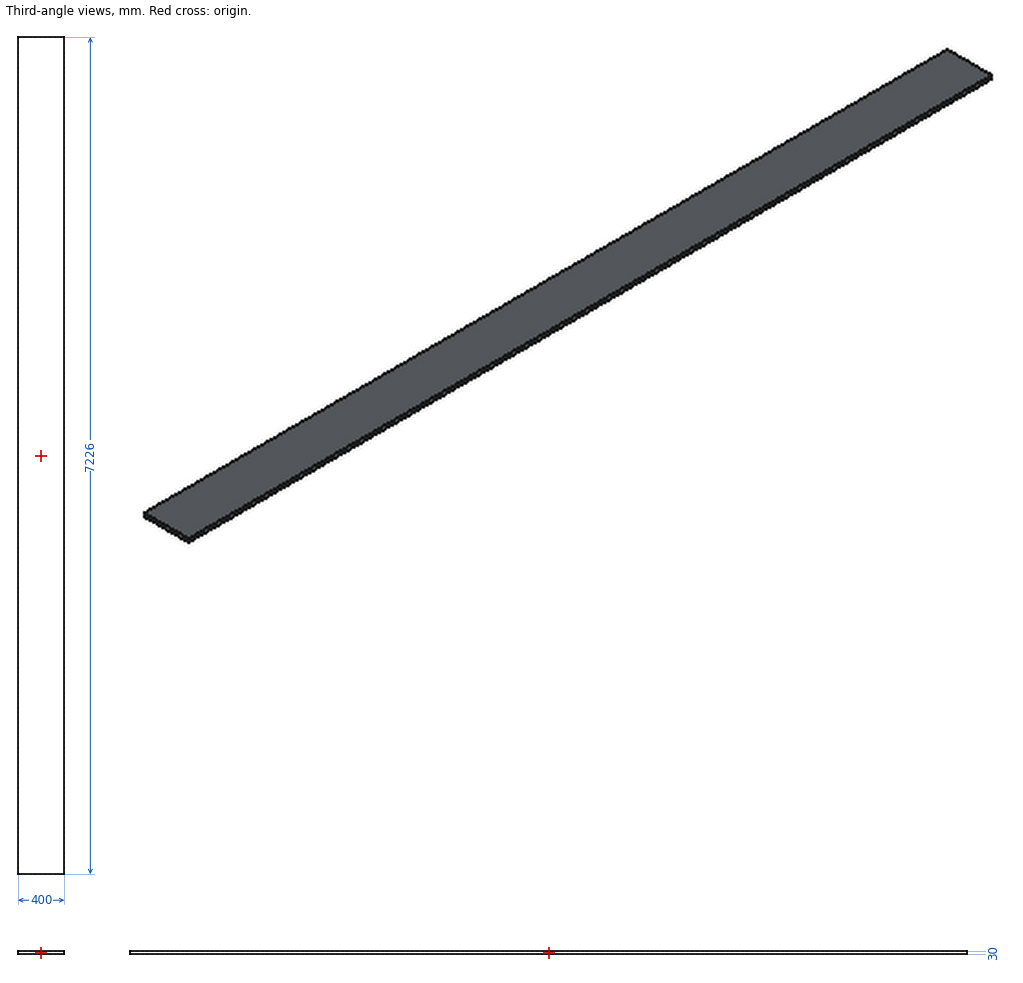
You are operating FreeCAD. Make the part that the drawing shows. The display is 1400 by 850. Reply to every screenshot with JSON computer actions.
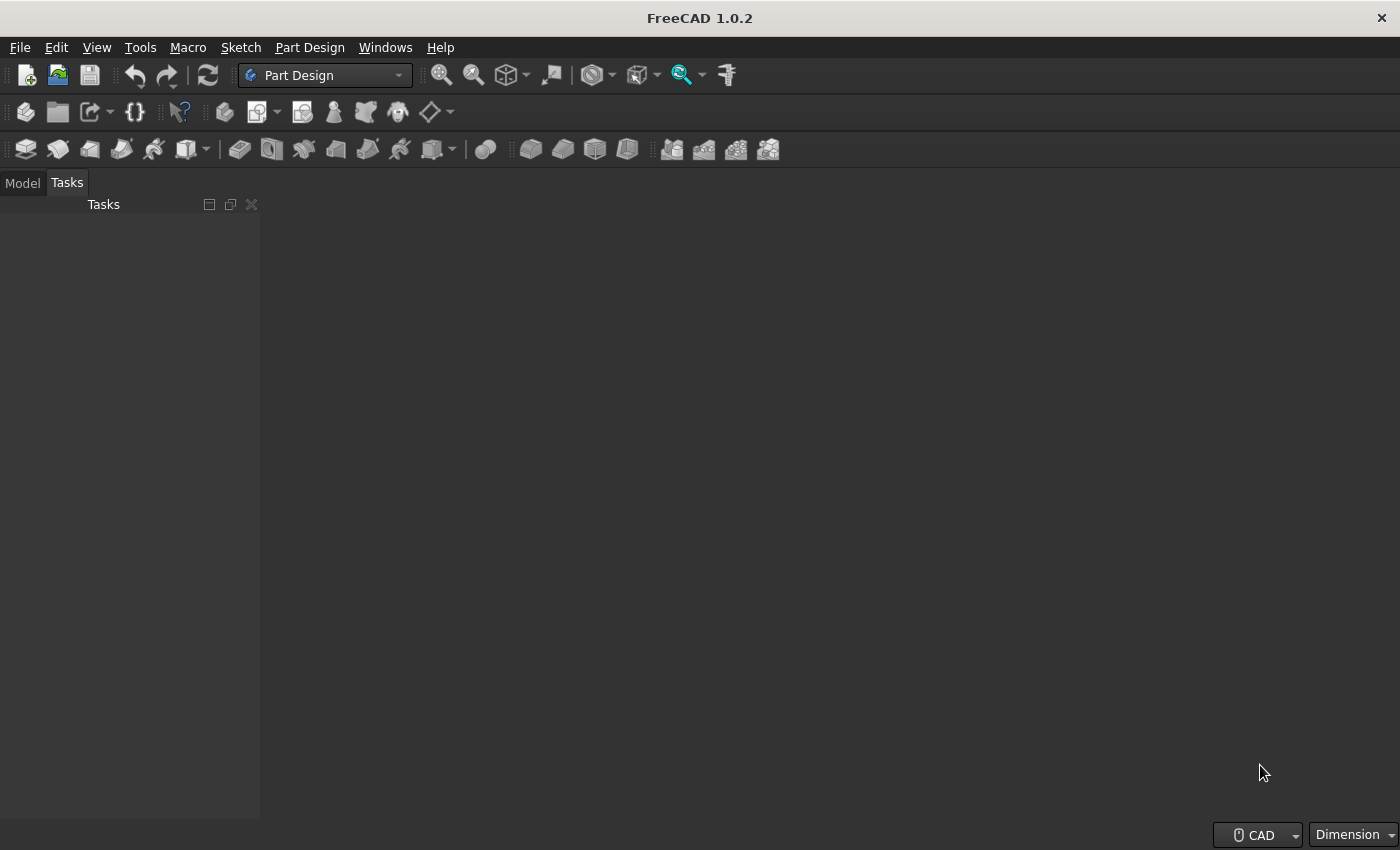
{"action": "left_click", "coordinate": [26, 76]}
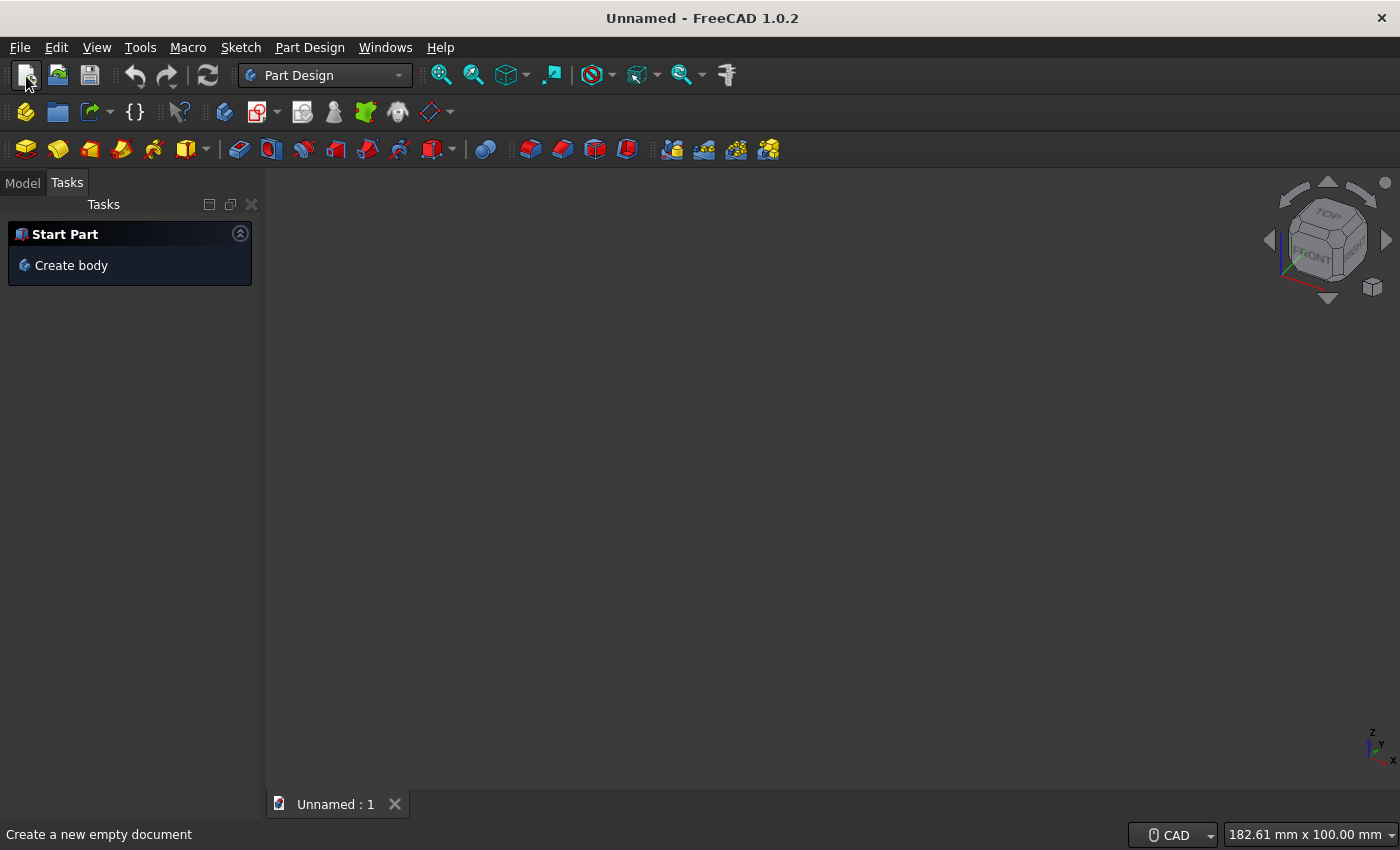
{"action": "left_click", "coordinate": [258, 112]}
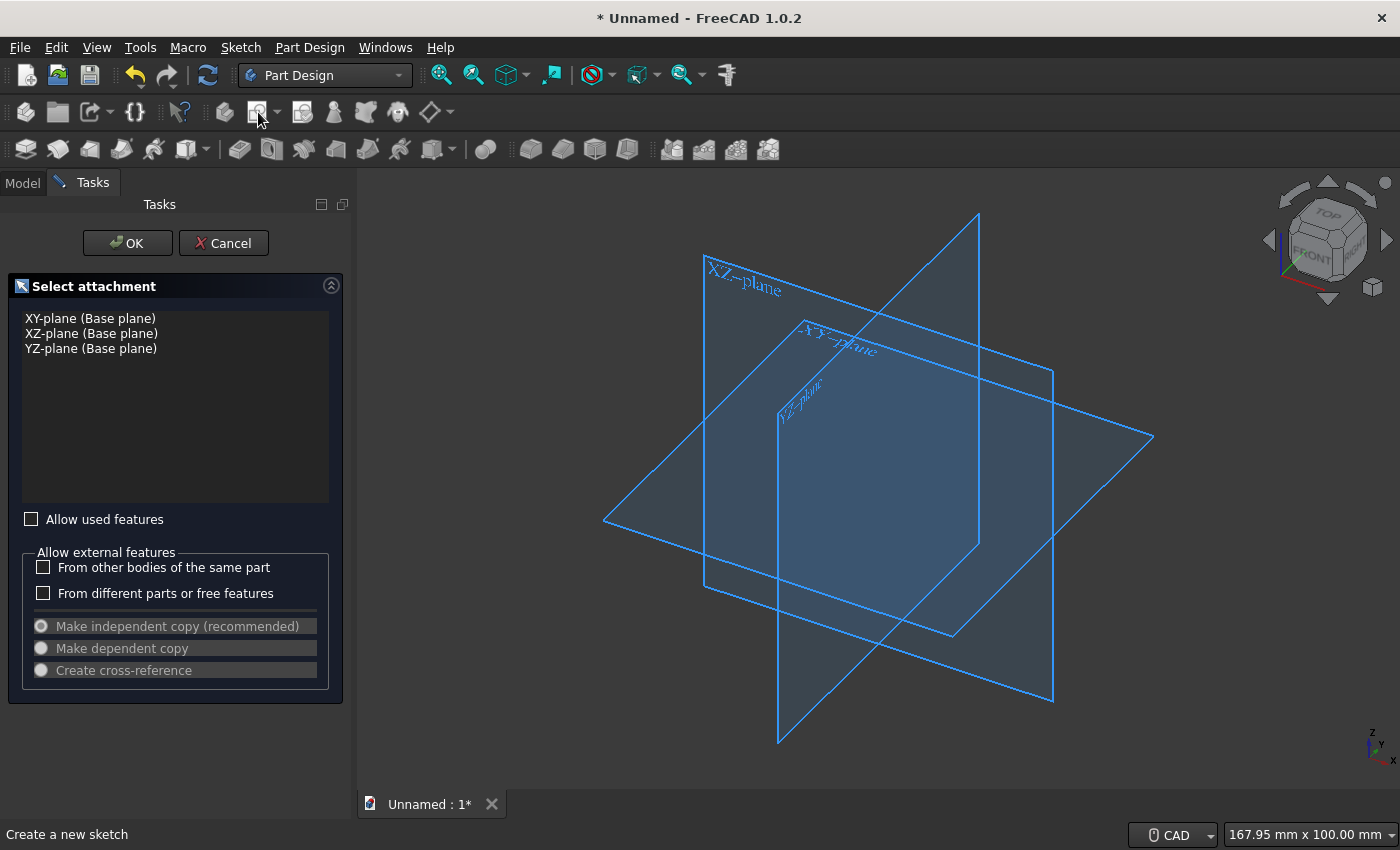
{"action": "left_click", "coordinate": [82, 318]}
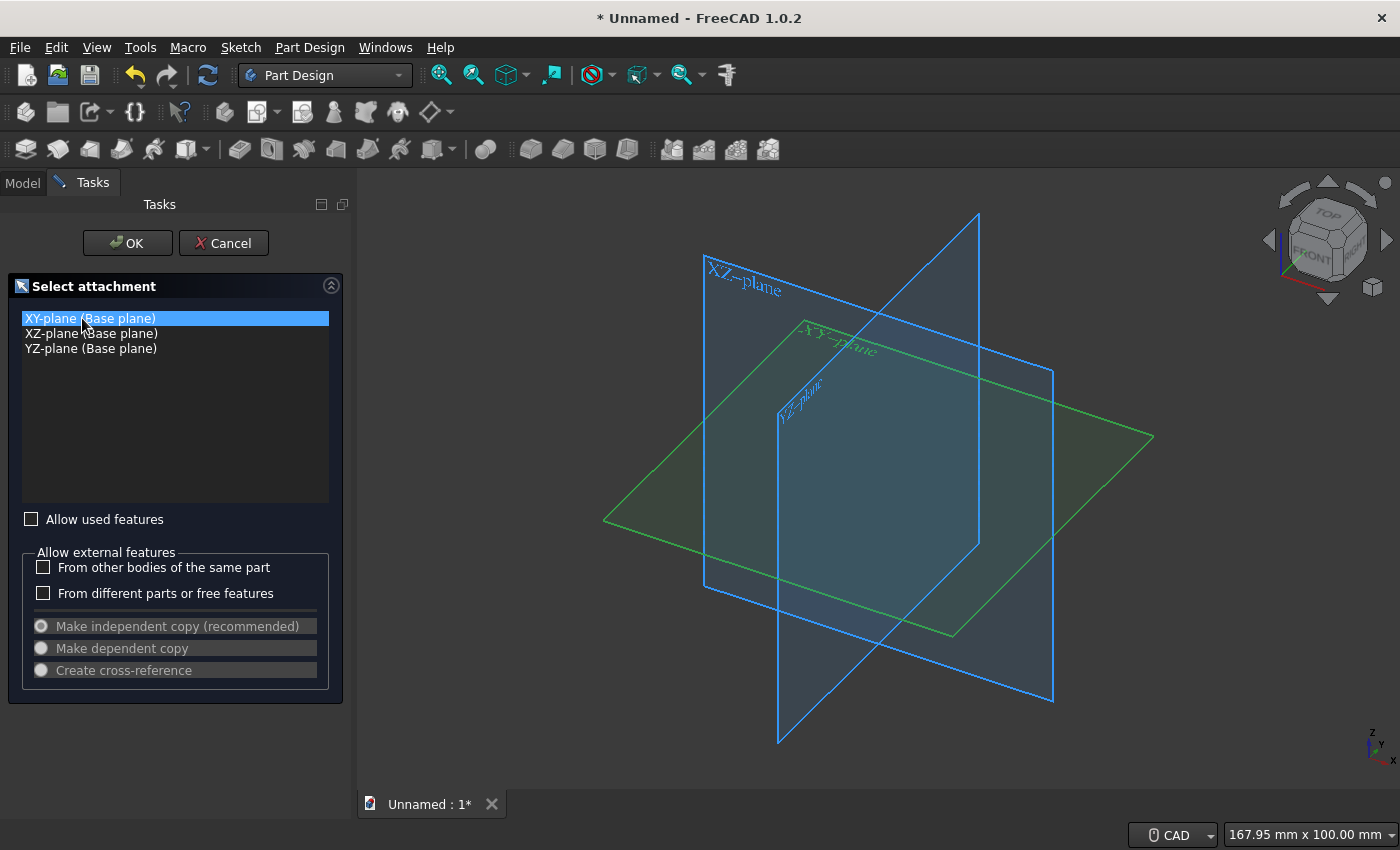
{"action": "left_click", "coordinate": [128, 243]}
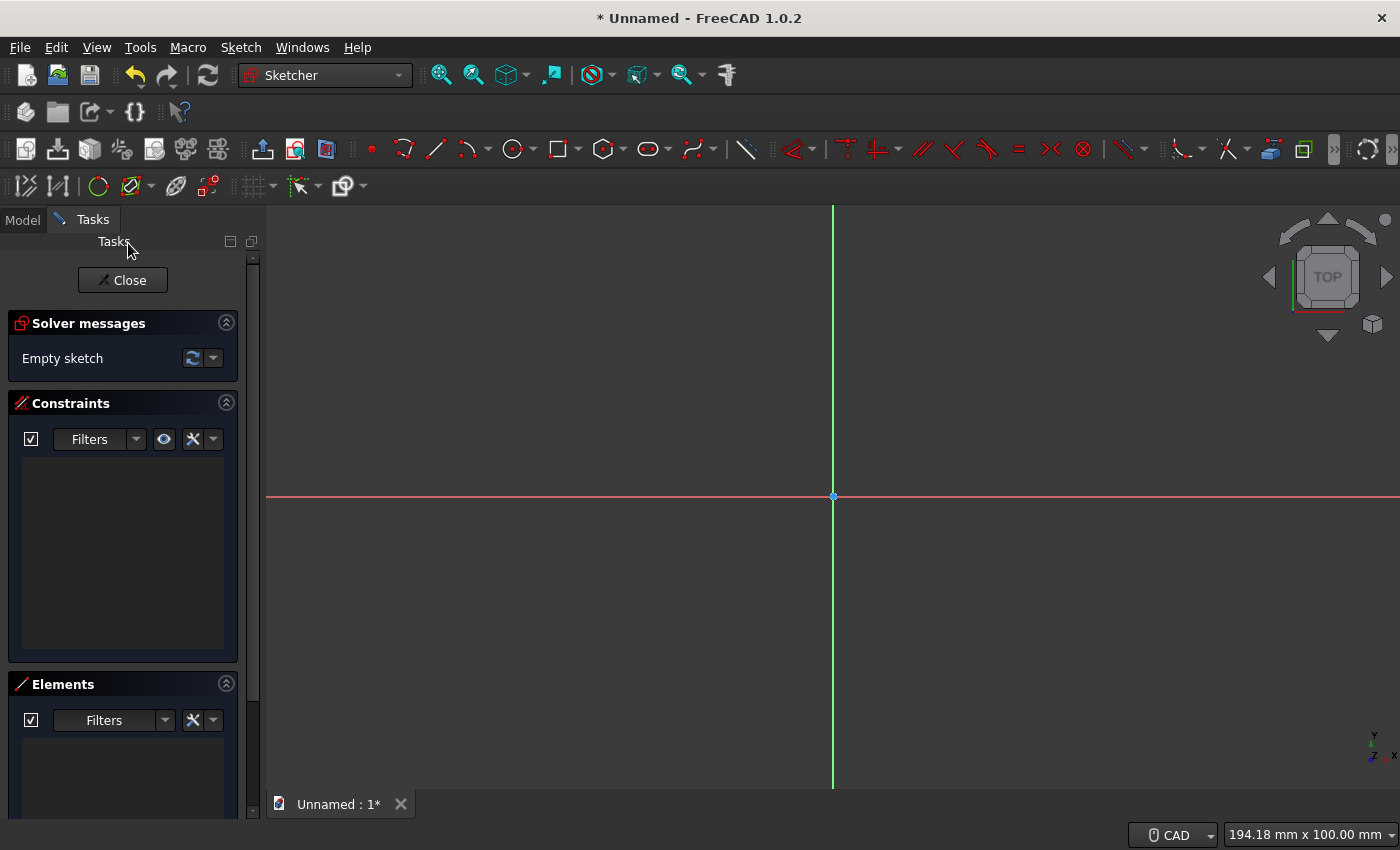
{"action": "scroll", "coordinate": [764, 497], "scroll_direction": "down", "scroll_amount": 15}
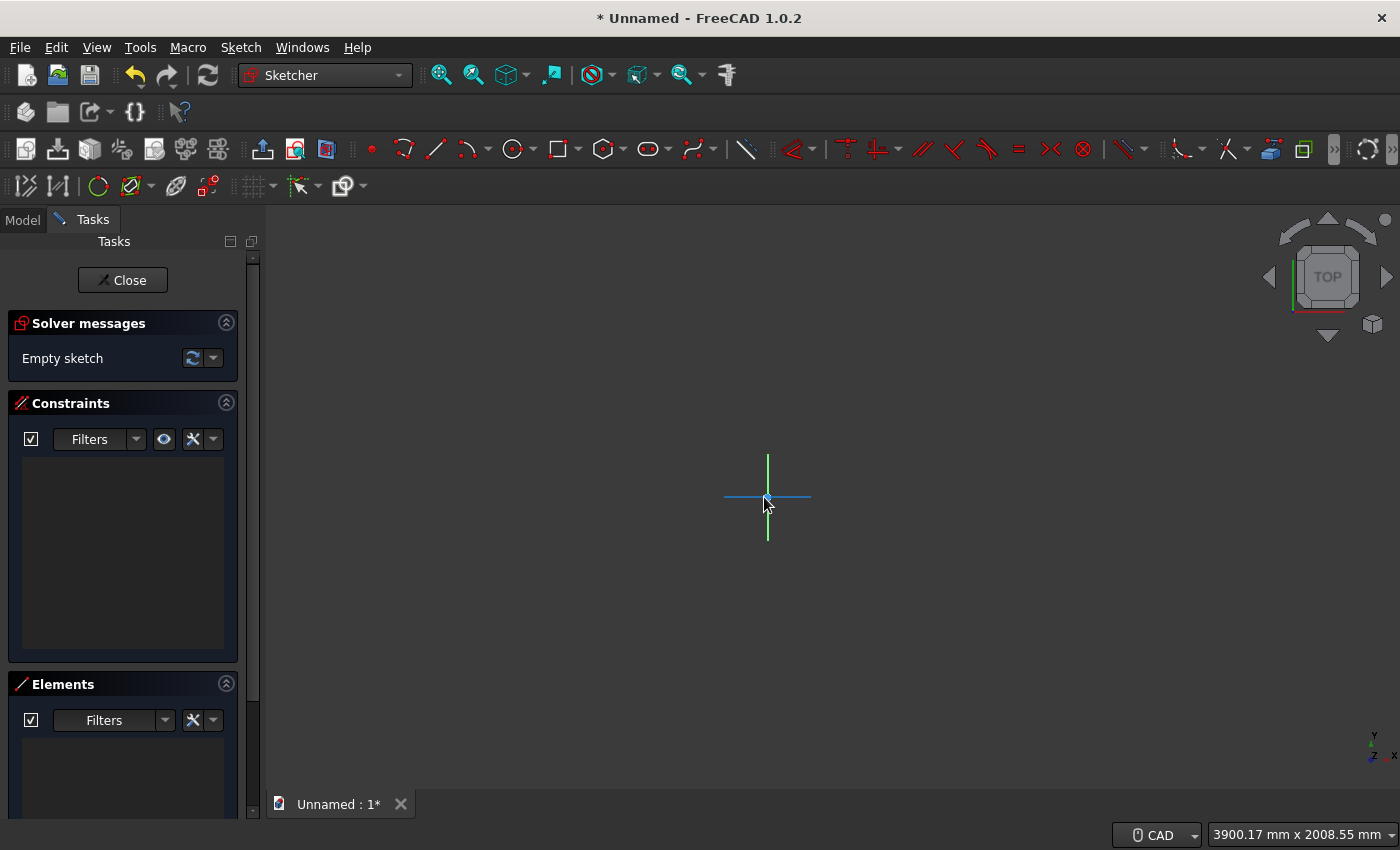
{"action": "scroll", "coordinate": [764, 497], "scroll_direction": "down", "scroll_amount": 9}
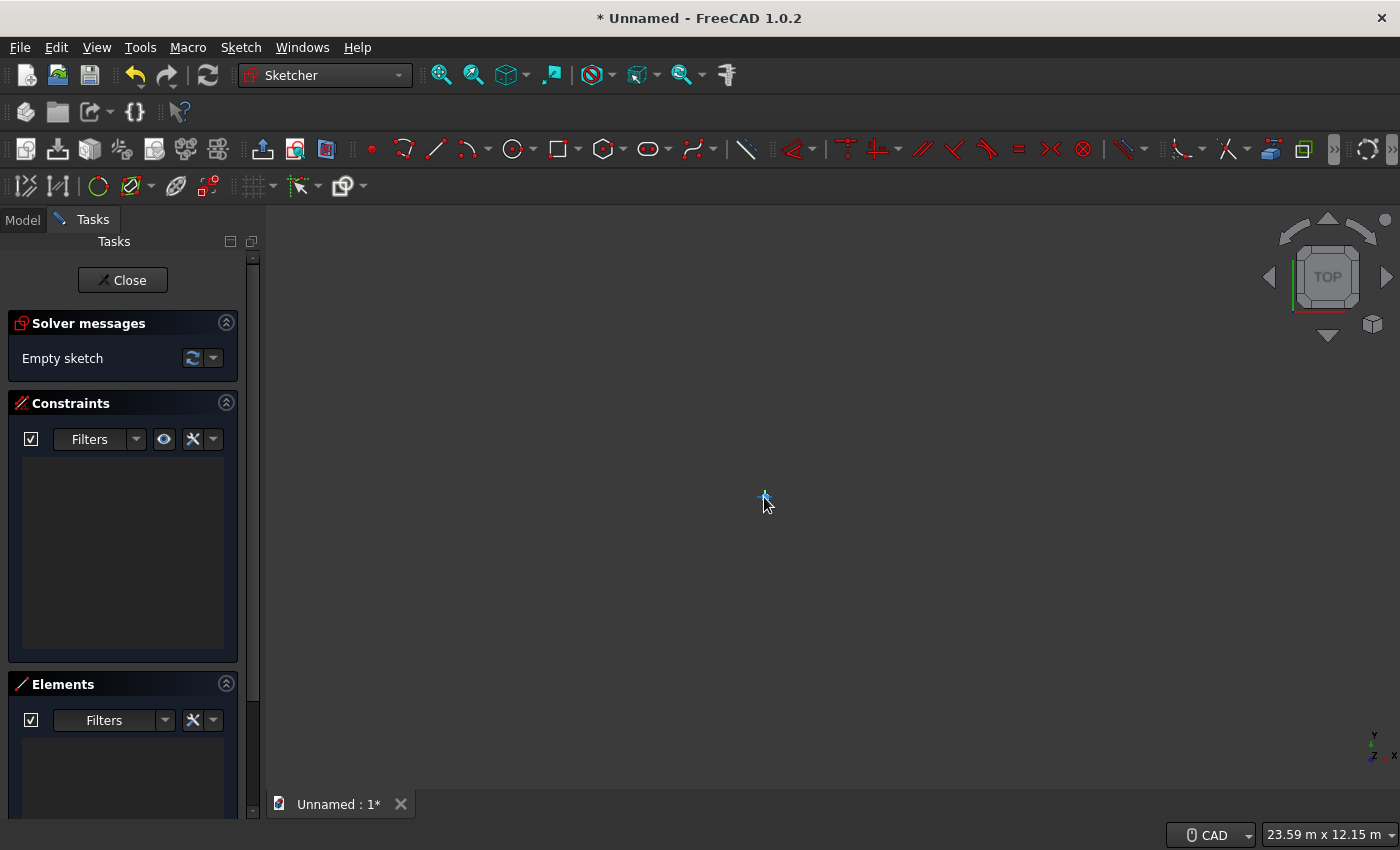
{"action": "left_click", "coordinate": [580, 150]}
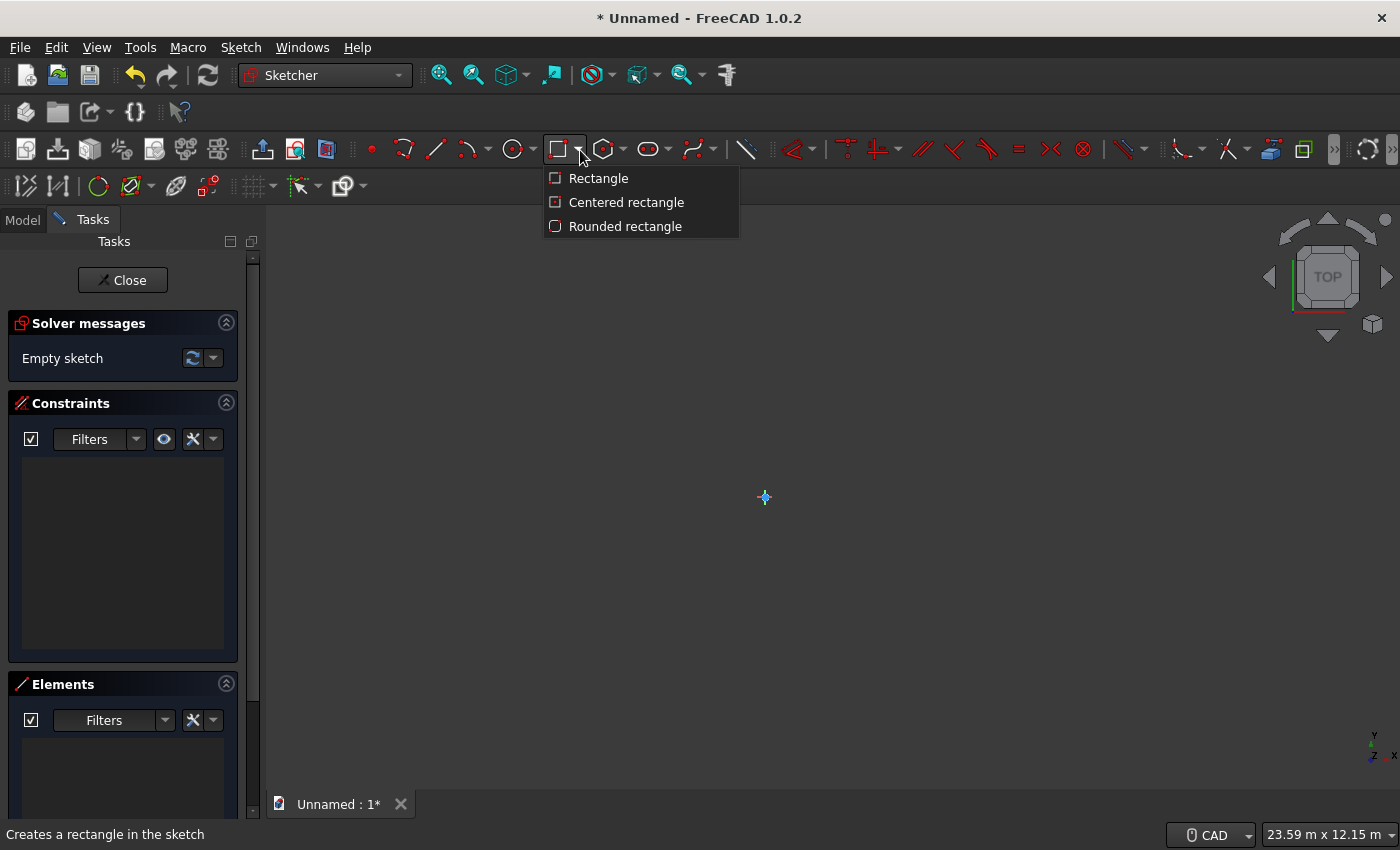
{"action": "left_click", "coordinate": [642, 202]}